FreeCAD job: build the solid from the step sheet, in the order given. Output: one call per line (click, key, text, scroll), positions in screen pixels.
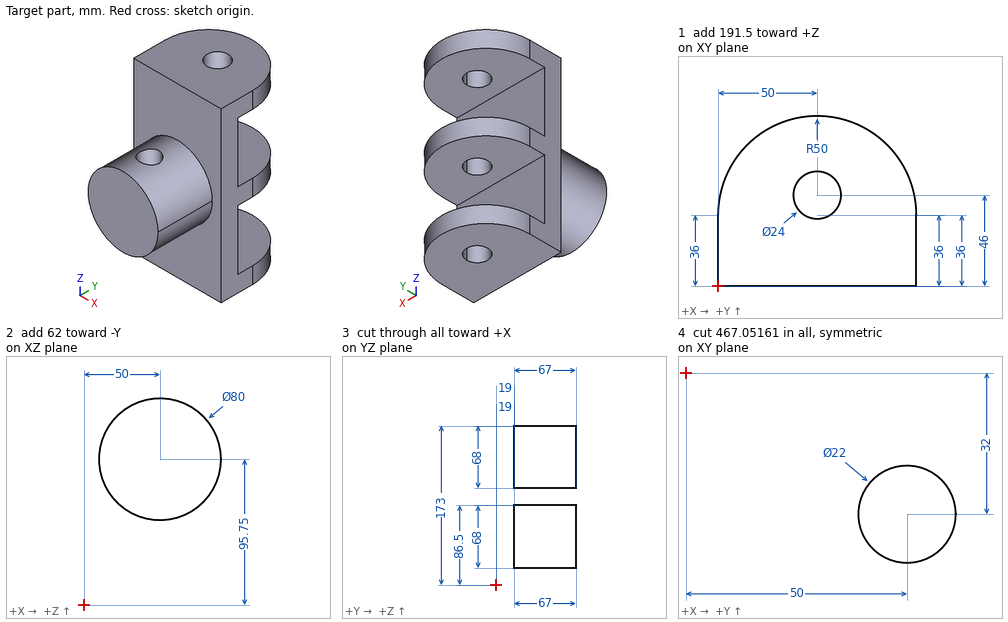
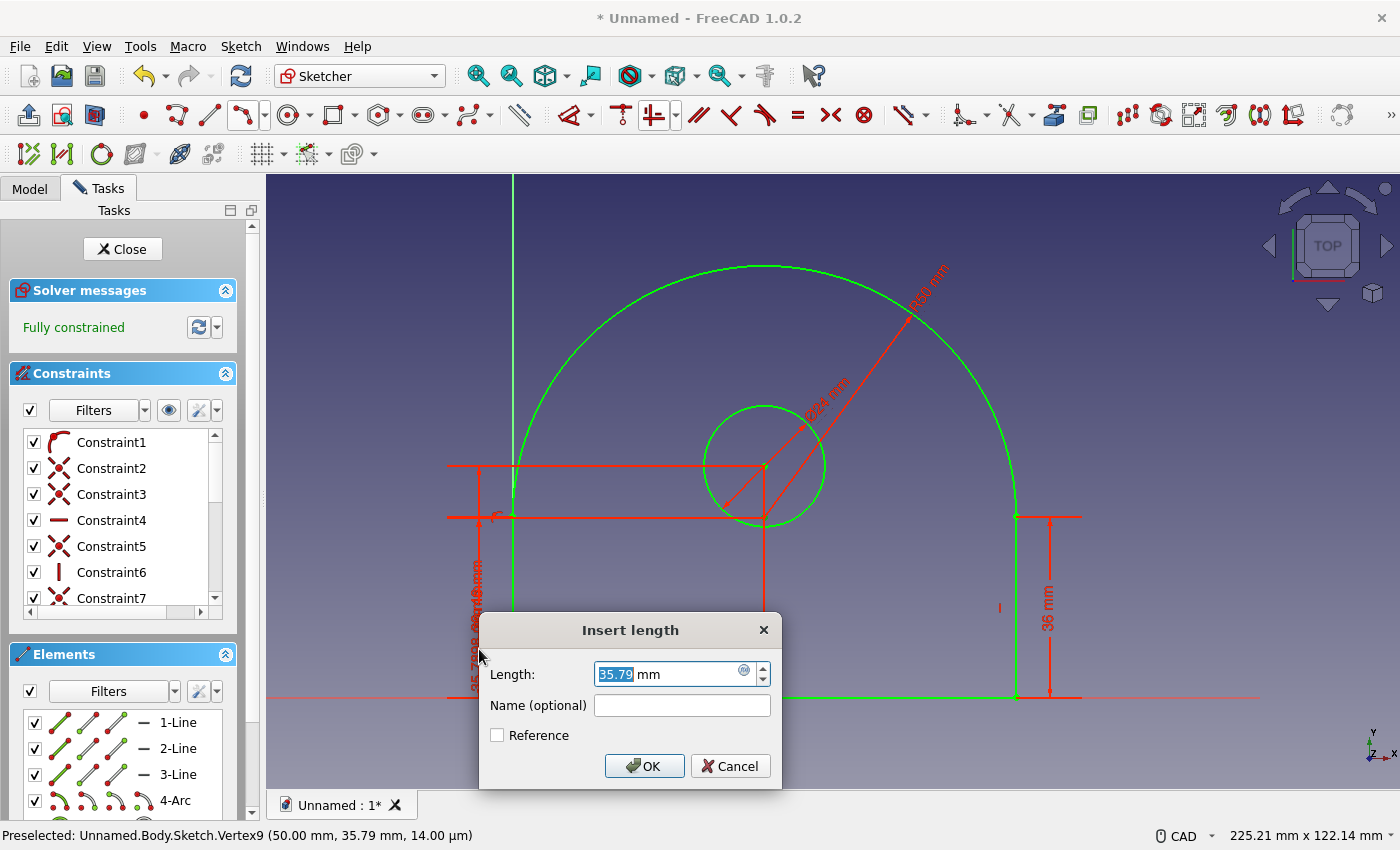
text(36)
key(Return)
key(Escape)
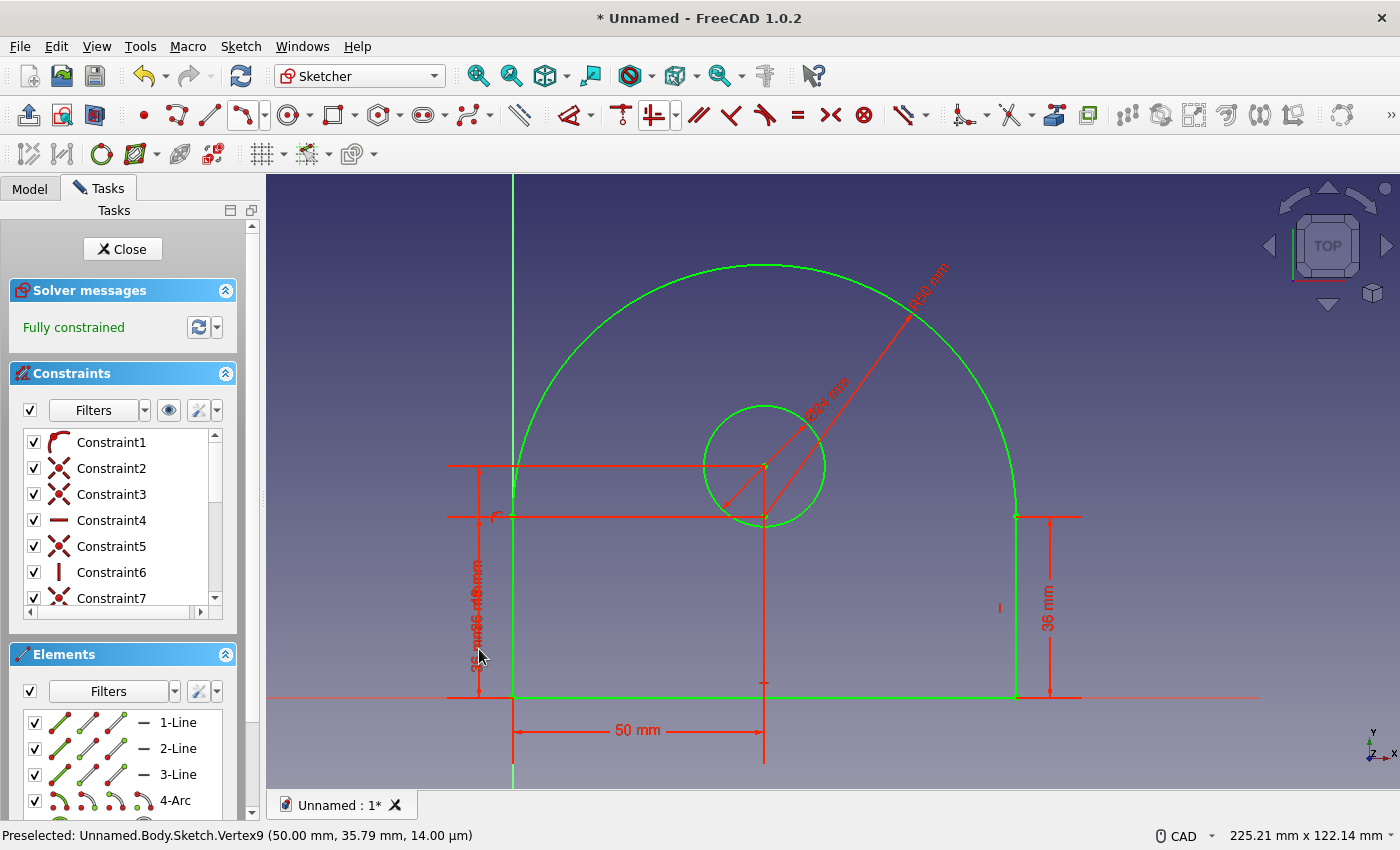
click(123, 249)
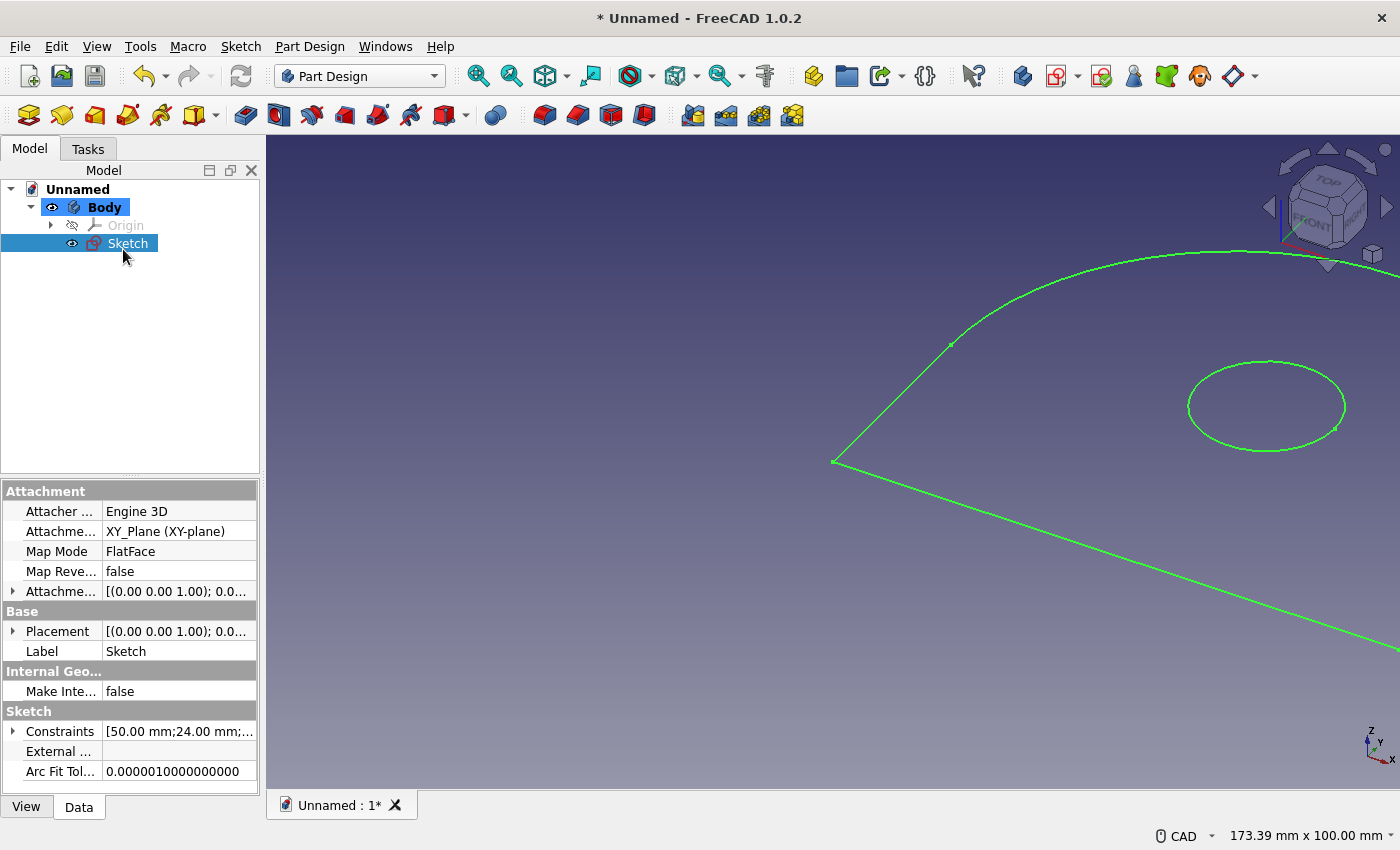
click(29, 116)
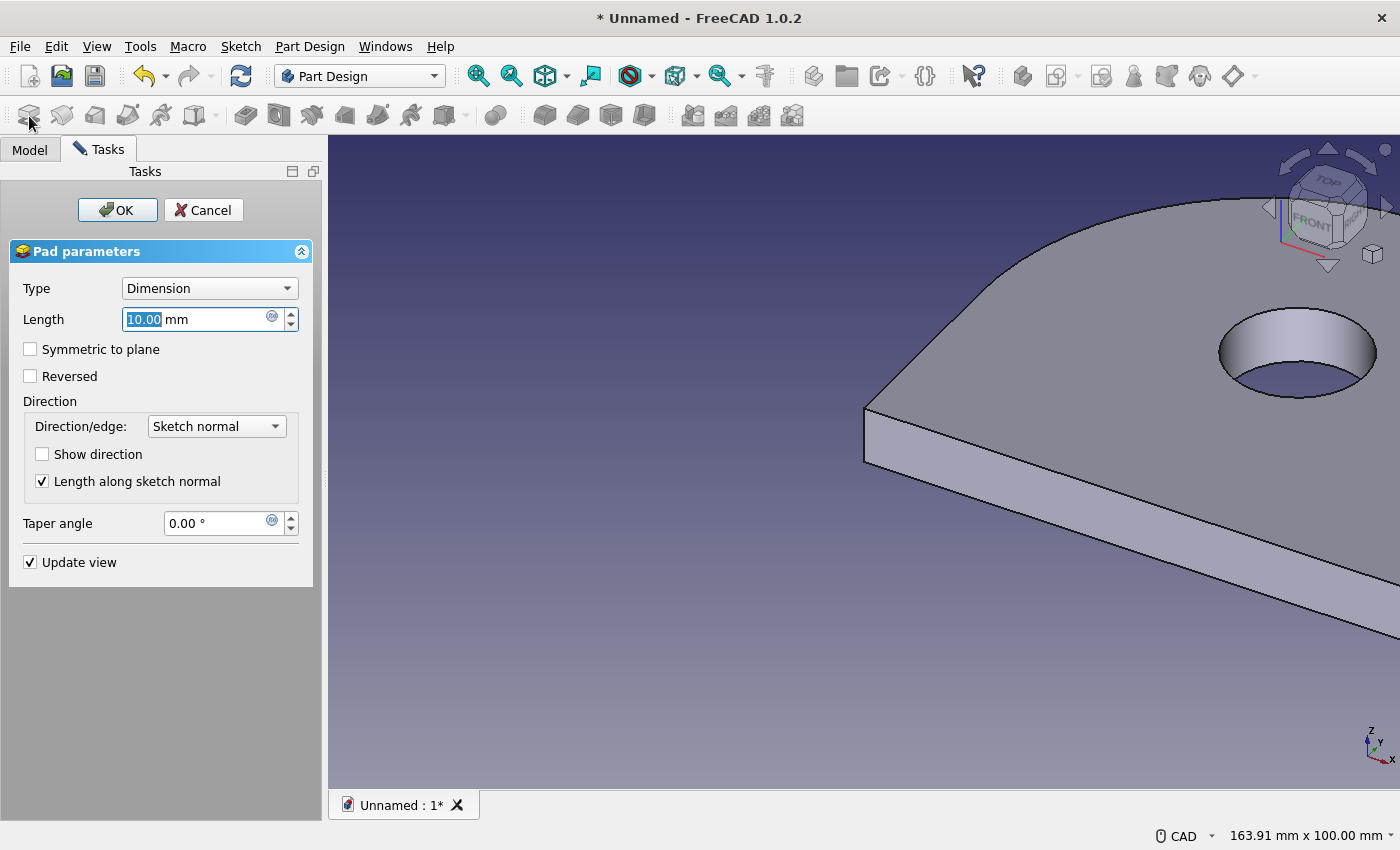
text(191.5)
key(Tab)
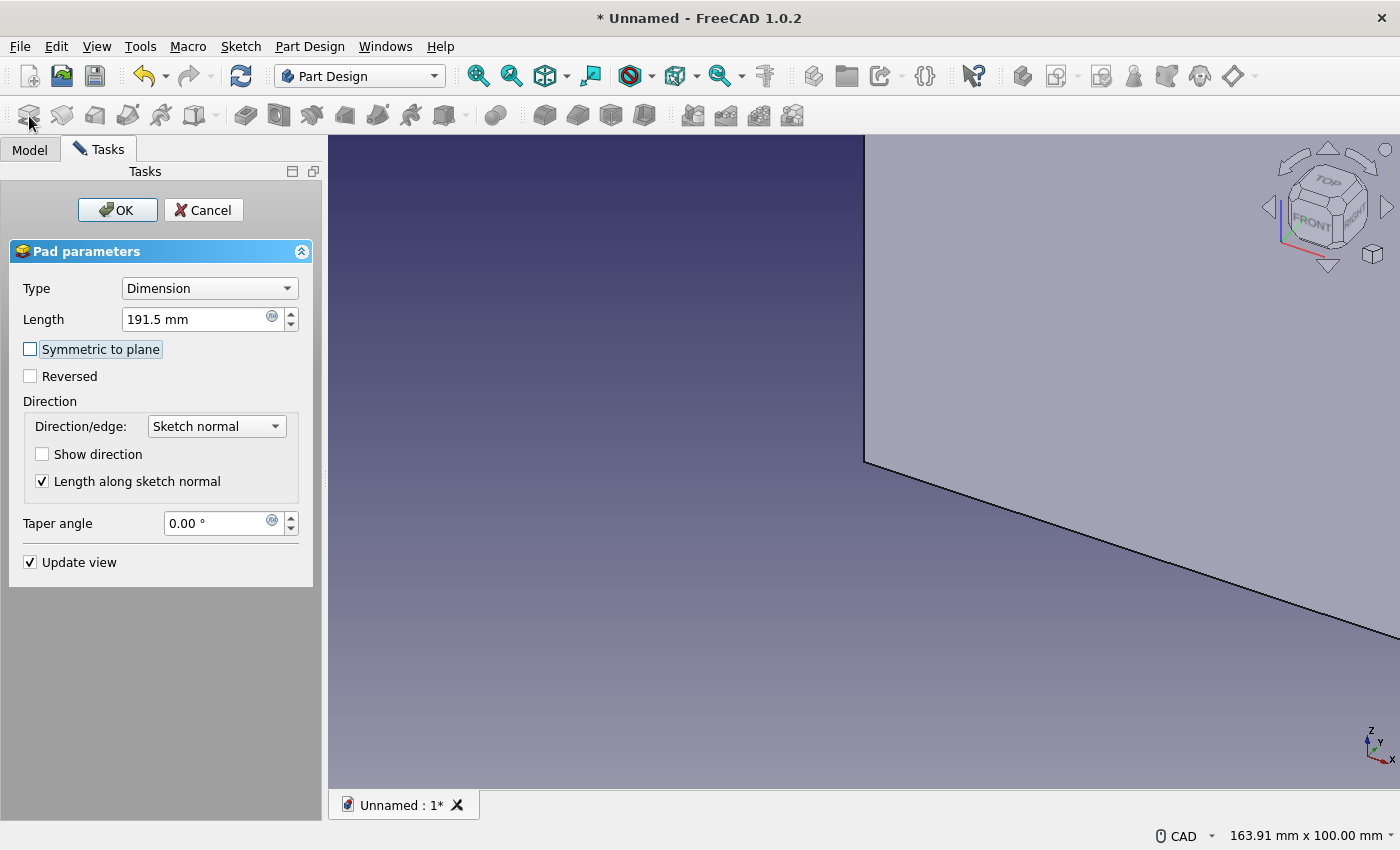
click(118, 210)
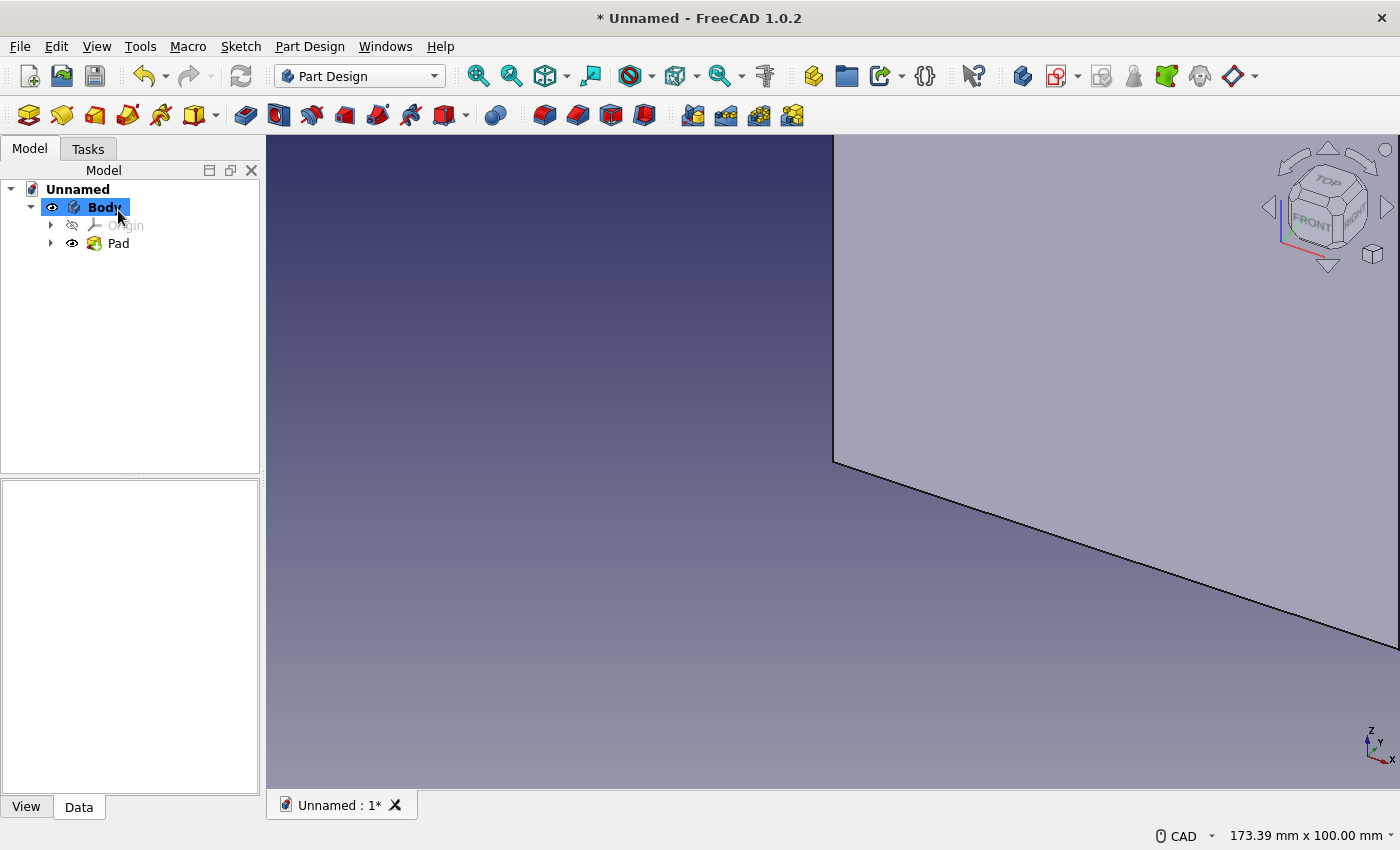
click(479, 76)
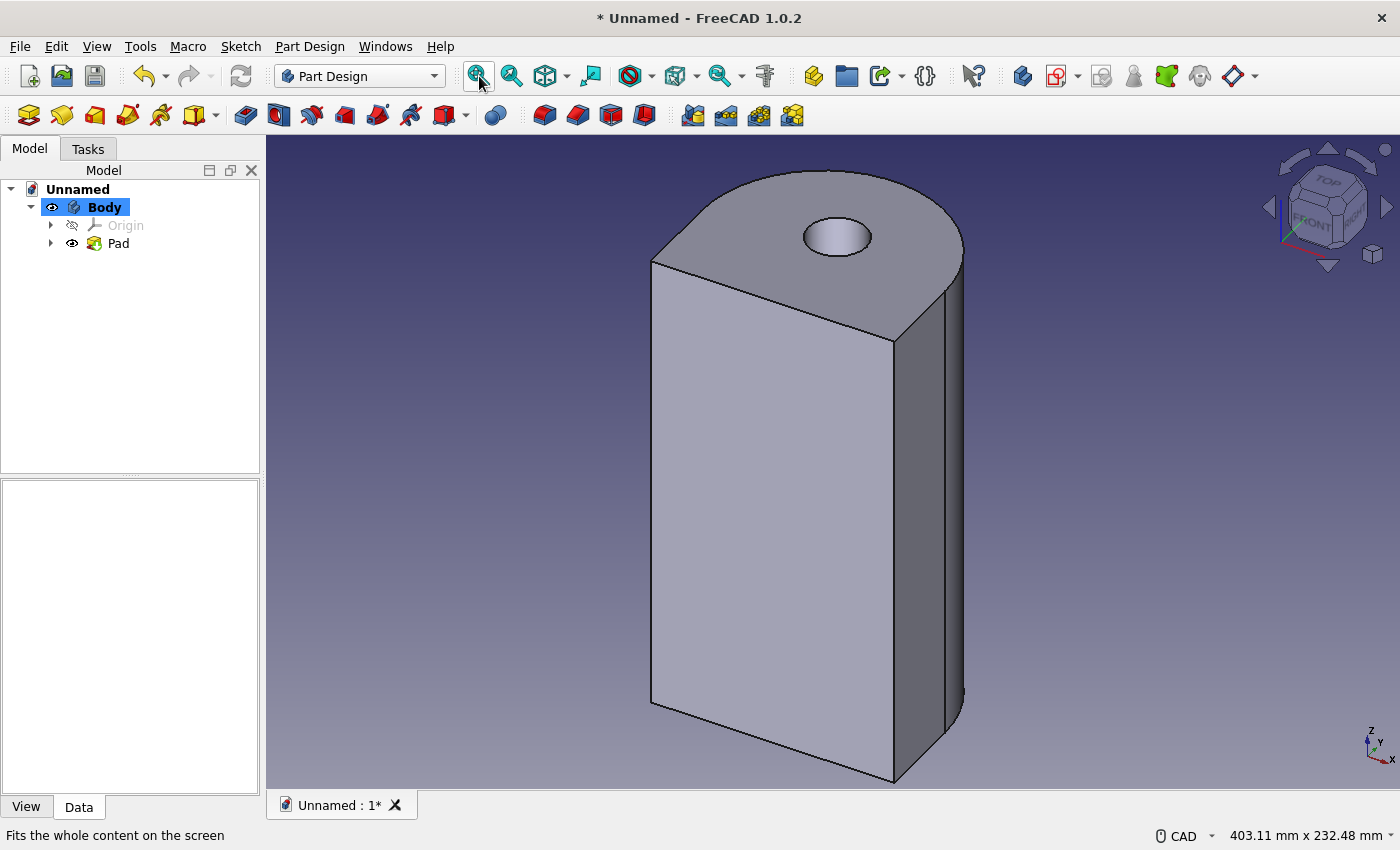
click(1056, 76)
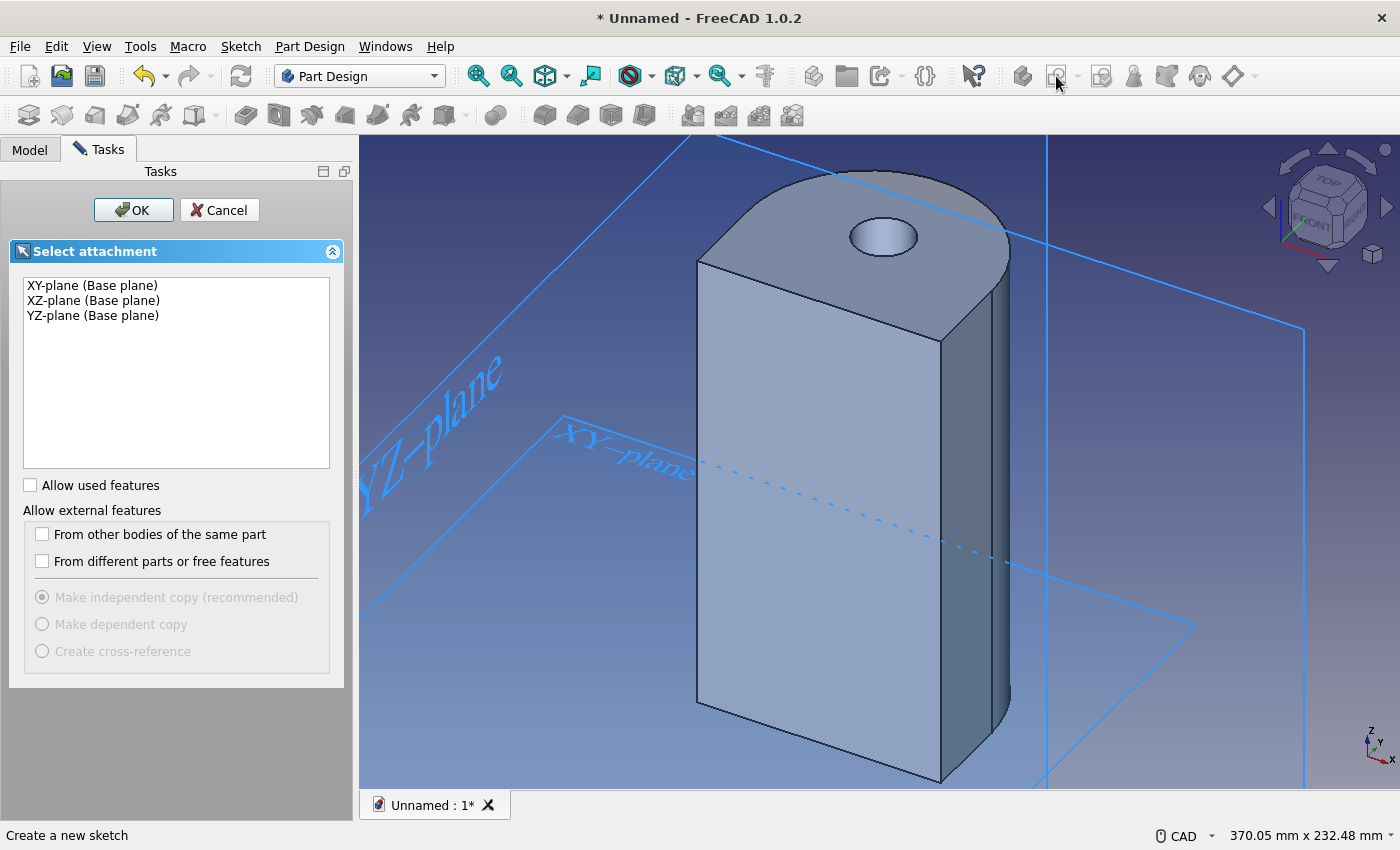
click(84, 300)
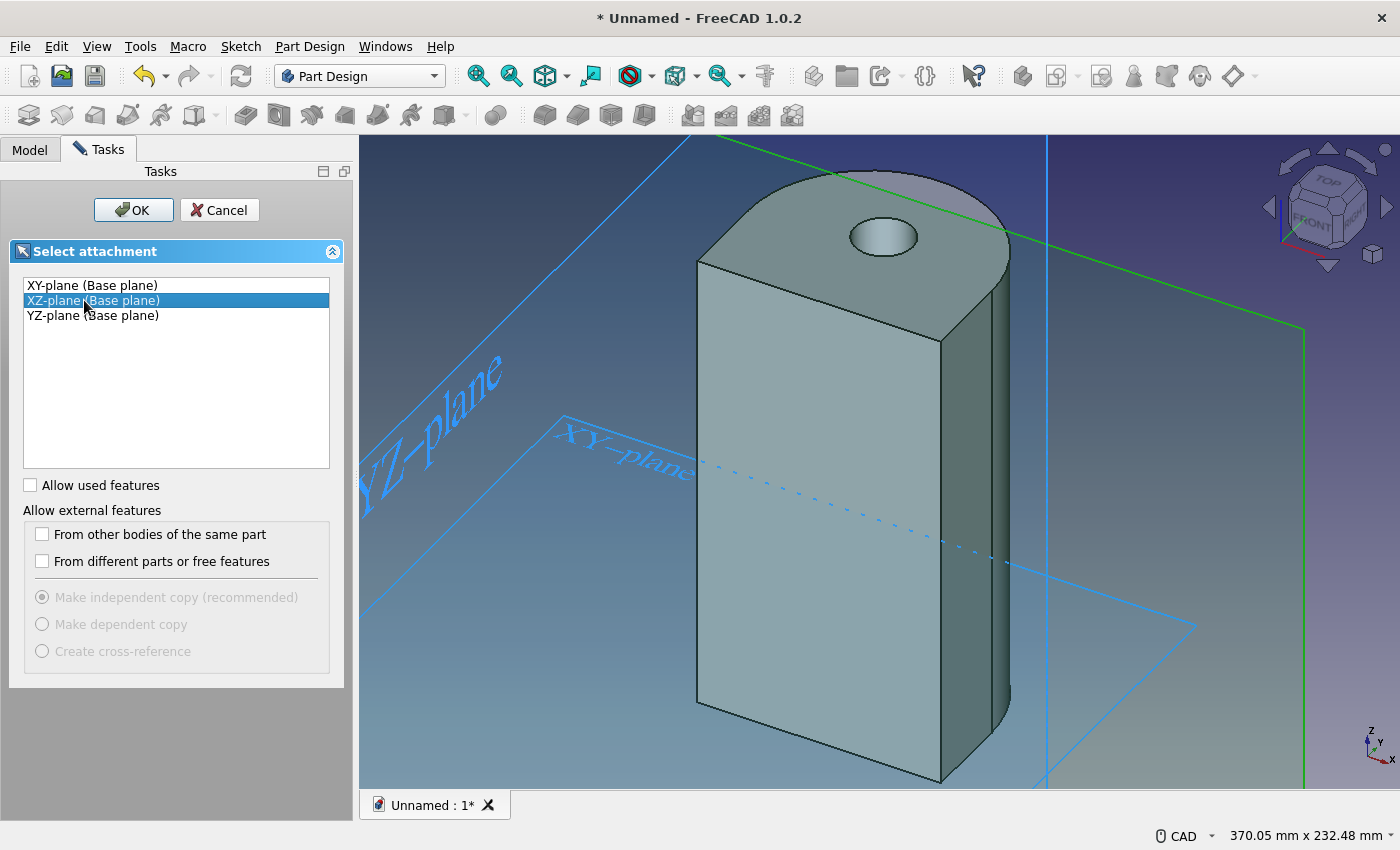
click(134, 210)